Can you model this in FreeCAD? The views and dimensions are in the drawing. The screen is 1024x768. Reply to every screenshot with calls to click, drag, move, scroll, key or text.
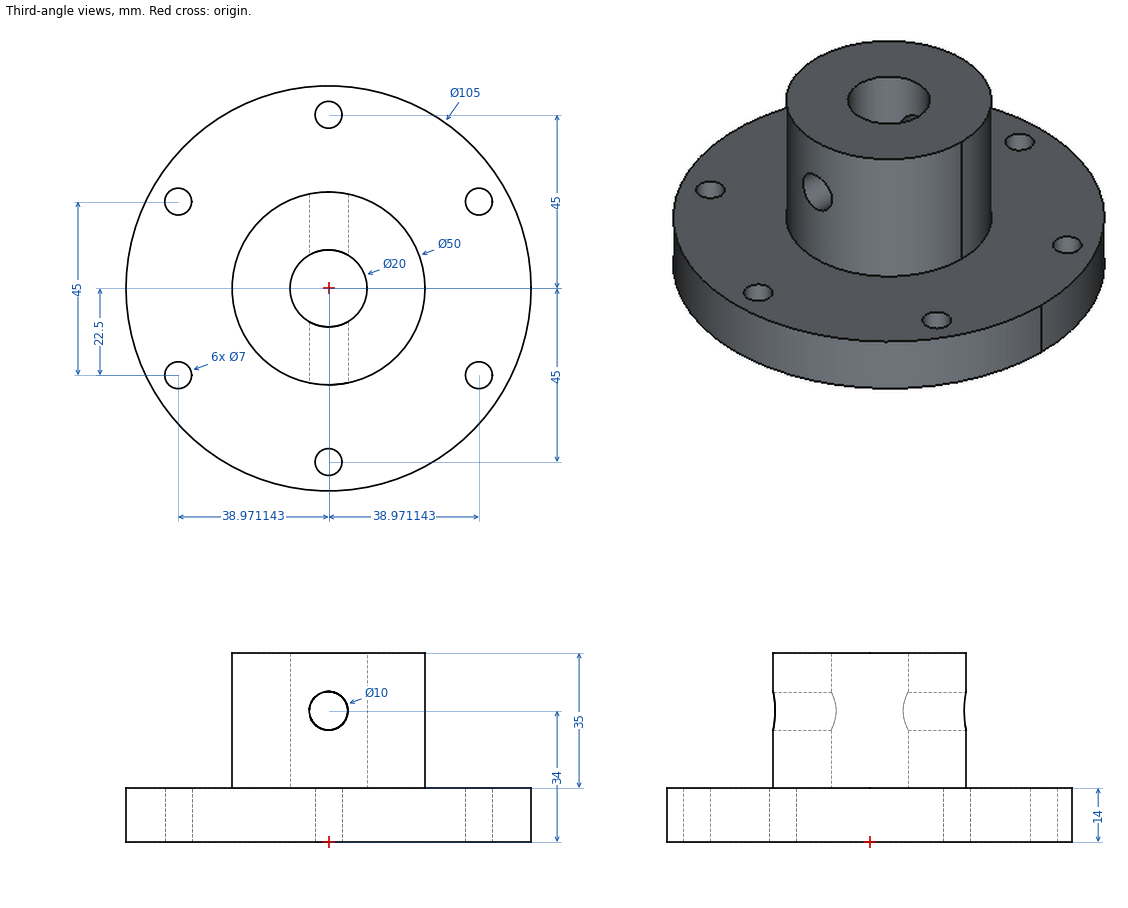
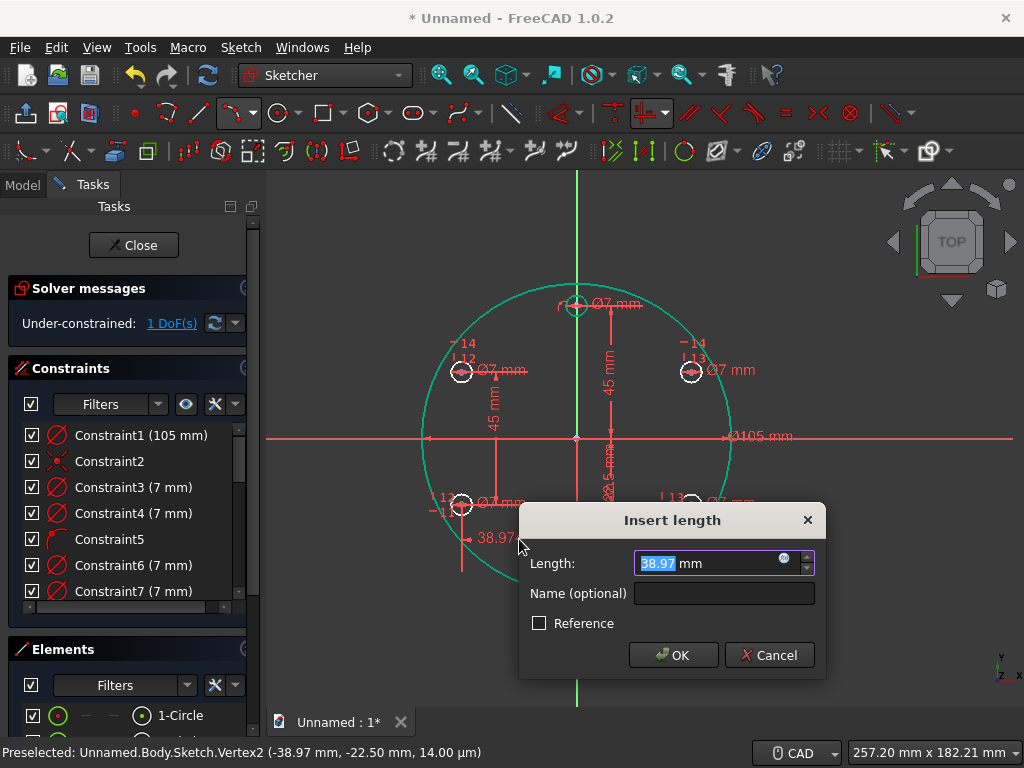
text(38.971143)
key(Return)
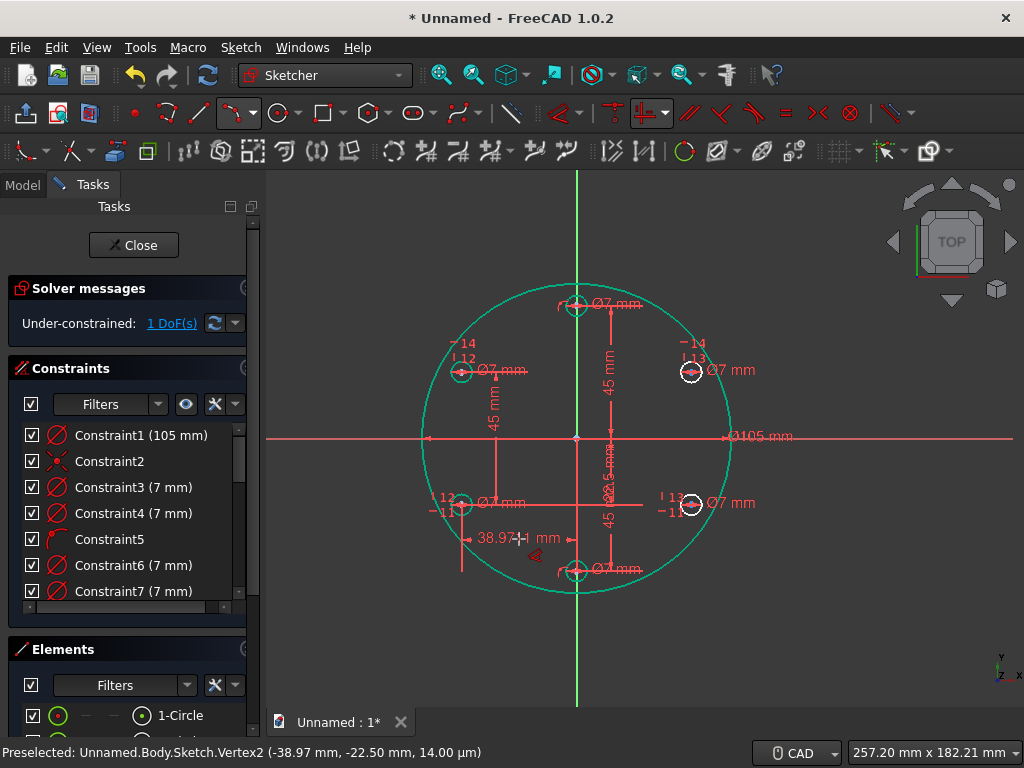
click(691, 505)
click(634, 539)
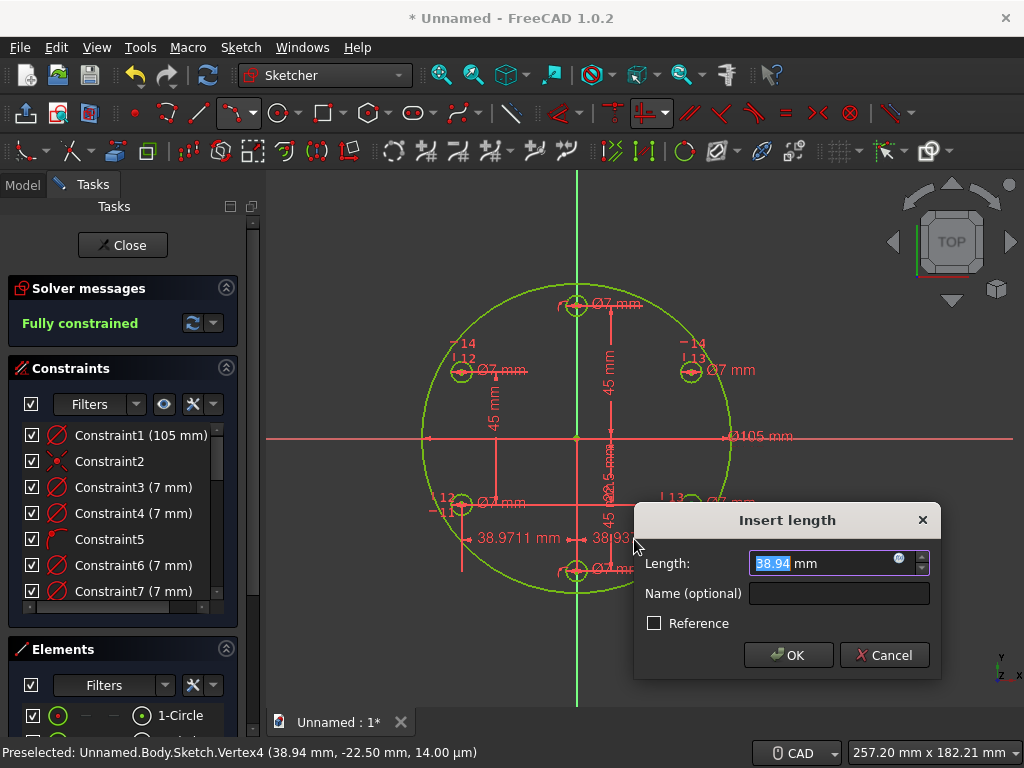
text(38.971143)
key(Return)
key(Escape)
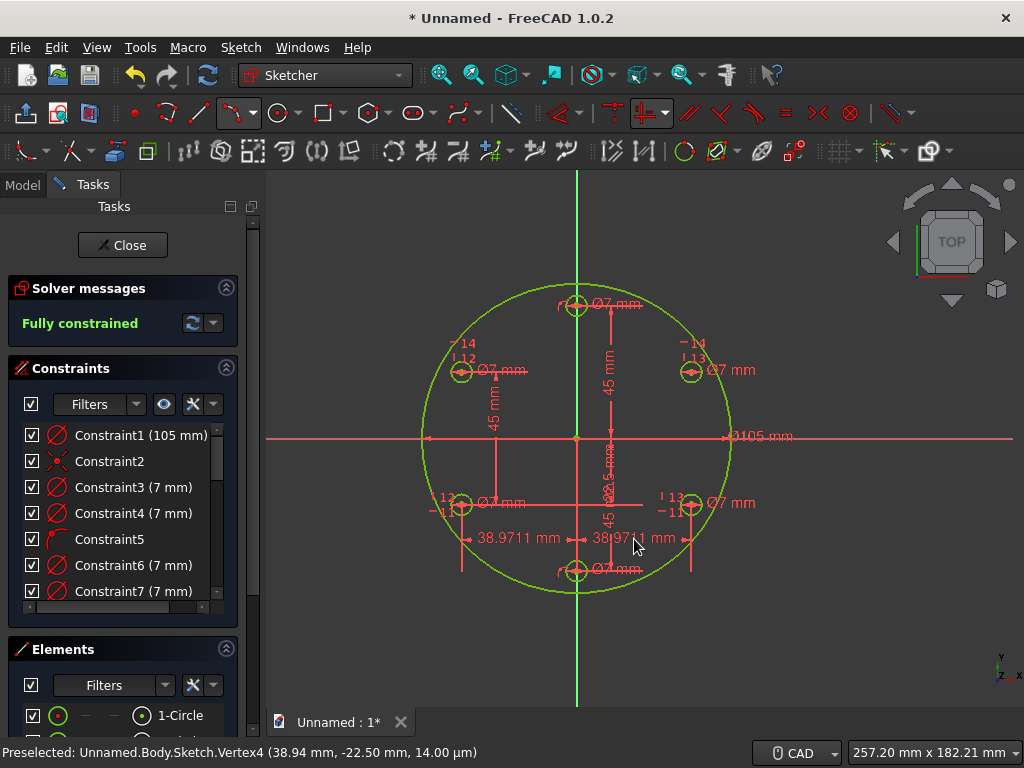
click(123, 245)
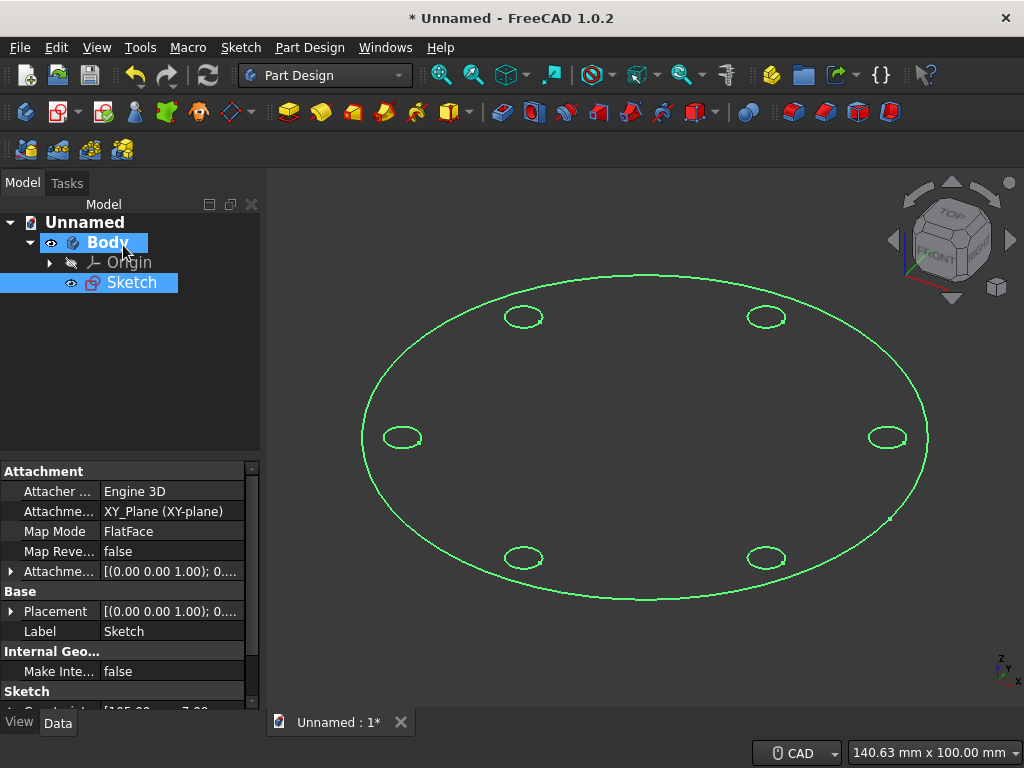
click(290, 112)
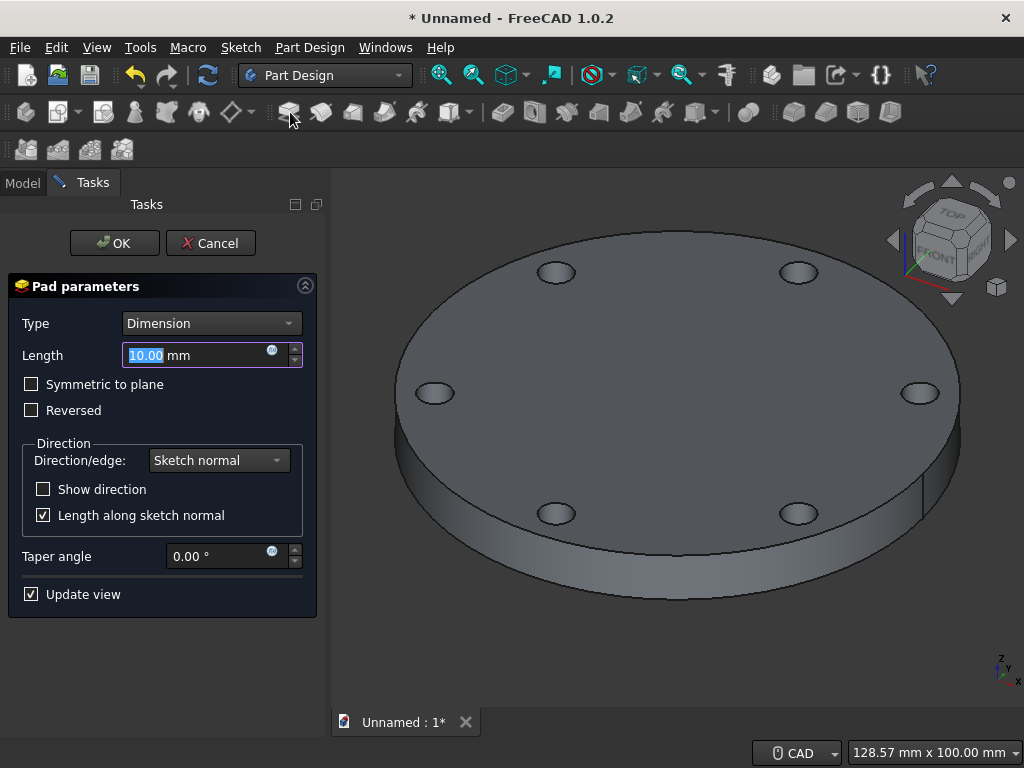
text(14)
key(Tab)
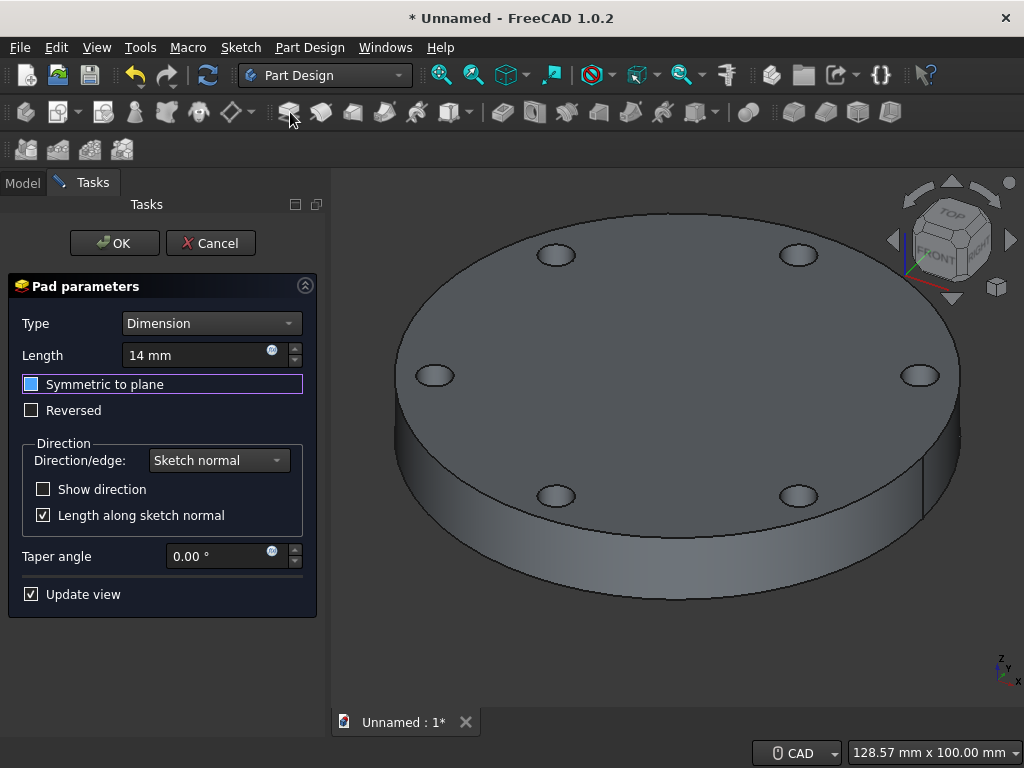
click(115, 243)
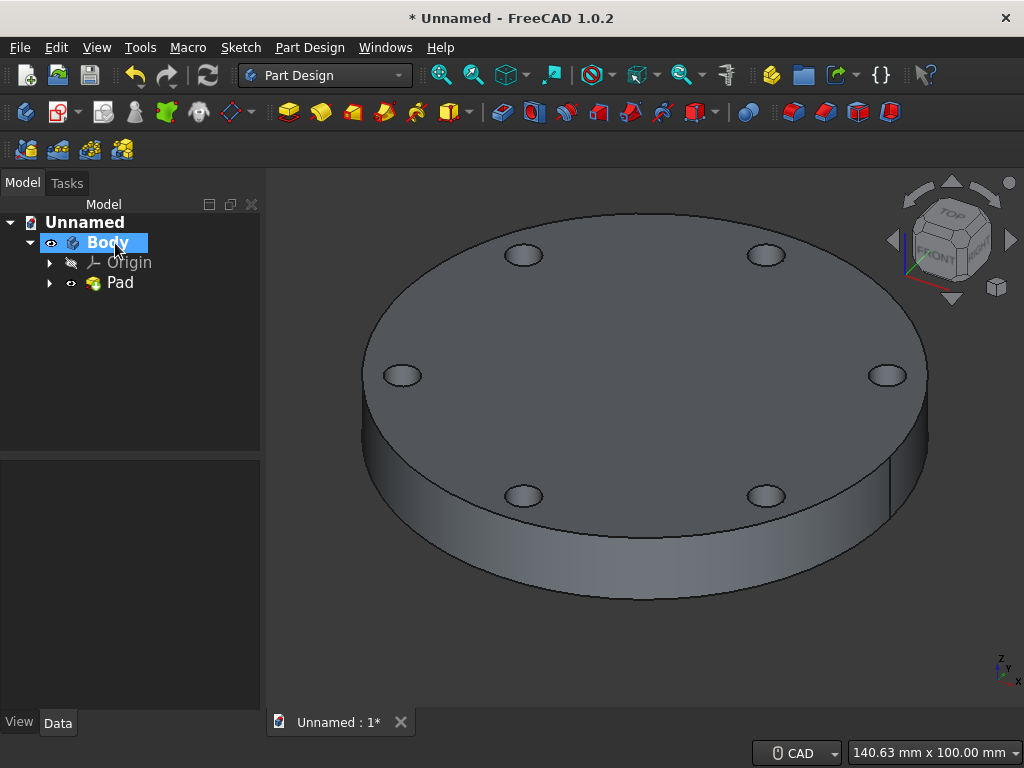
key(v)
key(f)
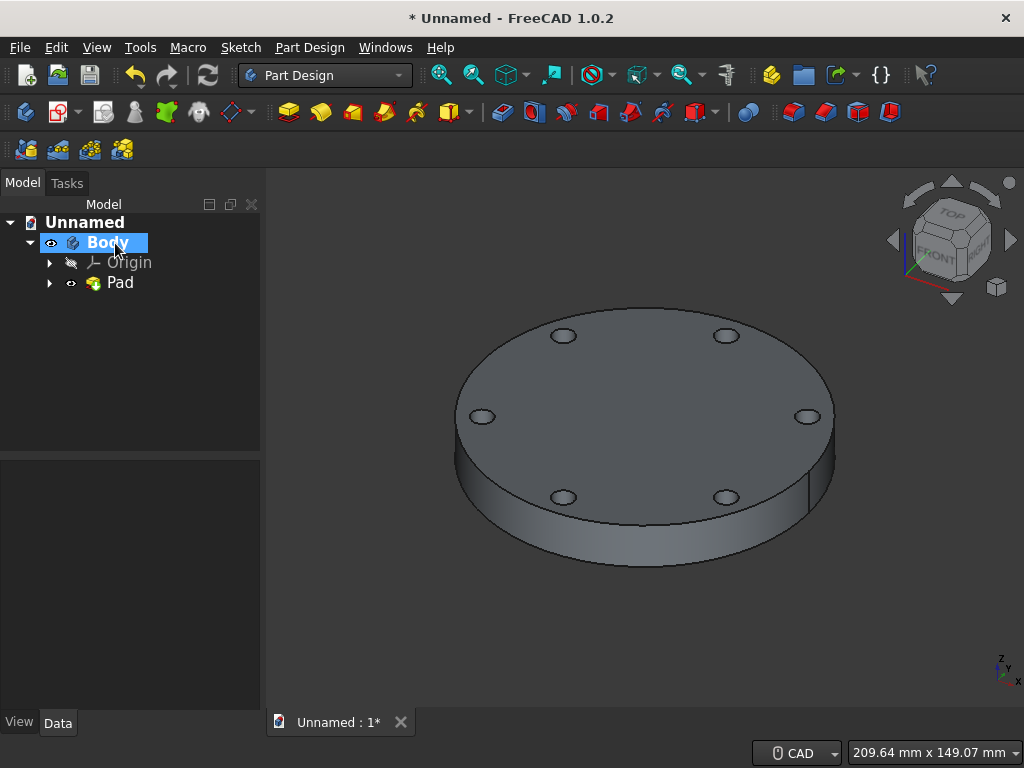
click(645, 416)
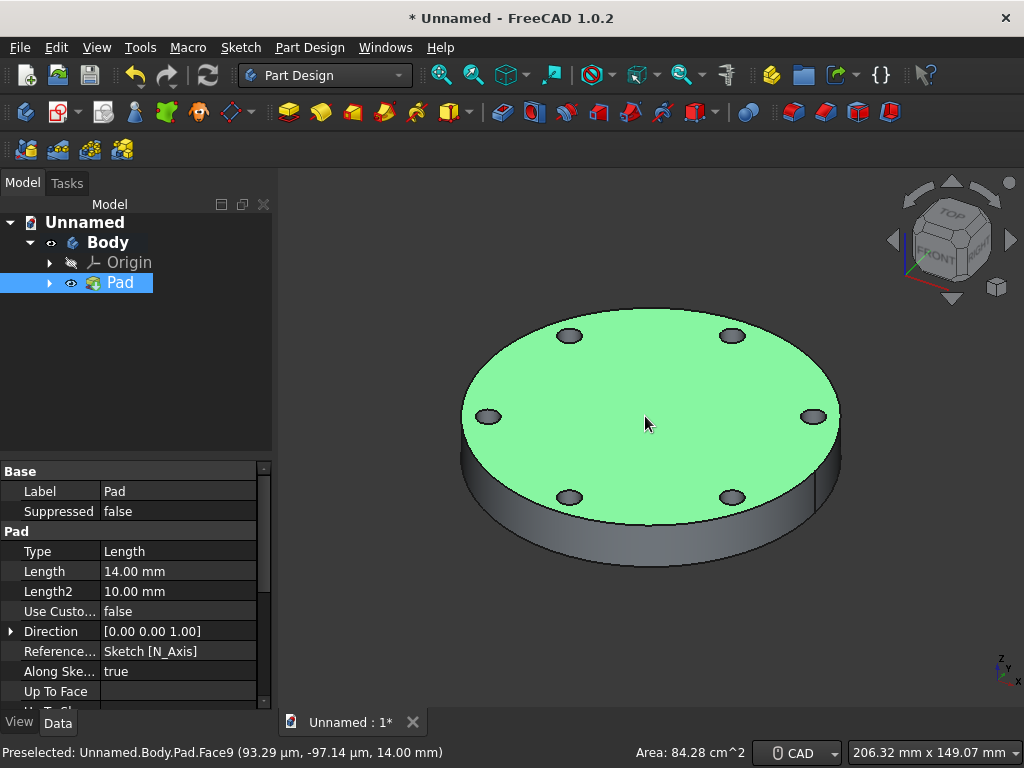
click(58, 112)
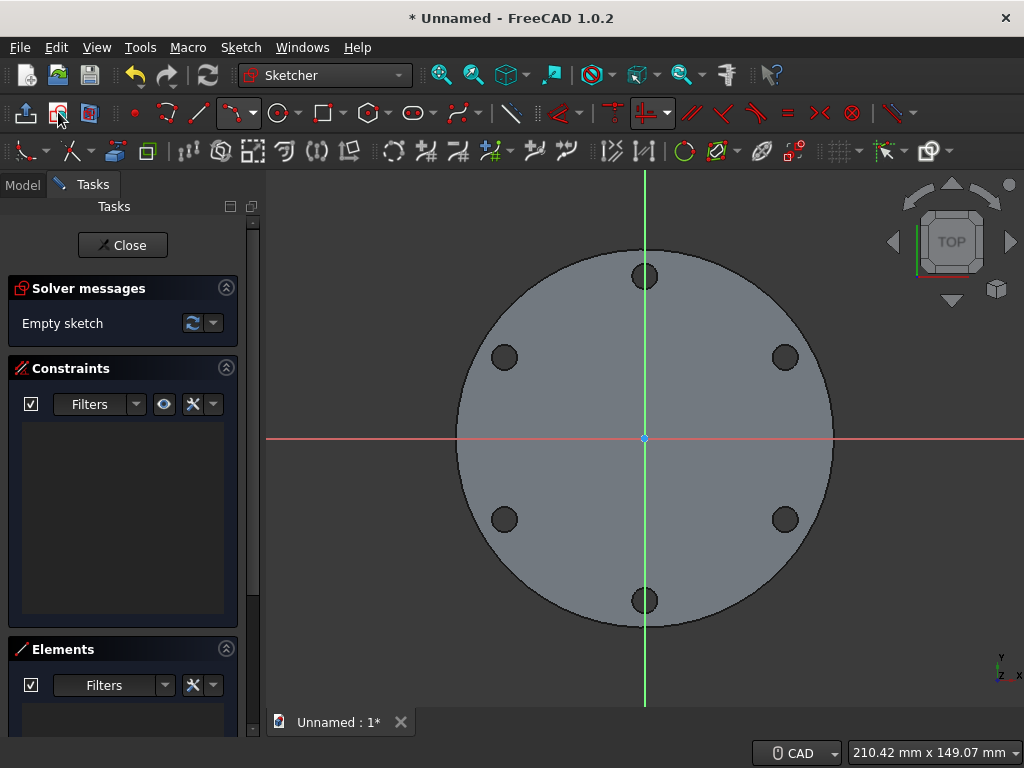
scroll(728, 438, up, 3)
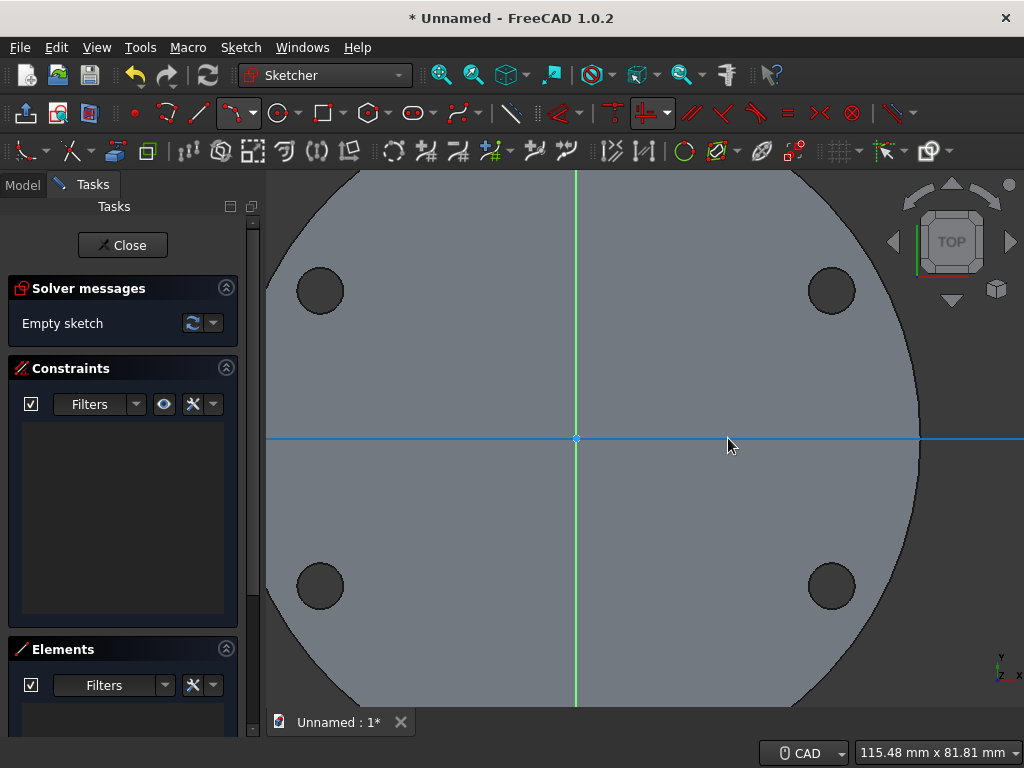
key(g)
key(c)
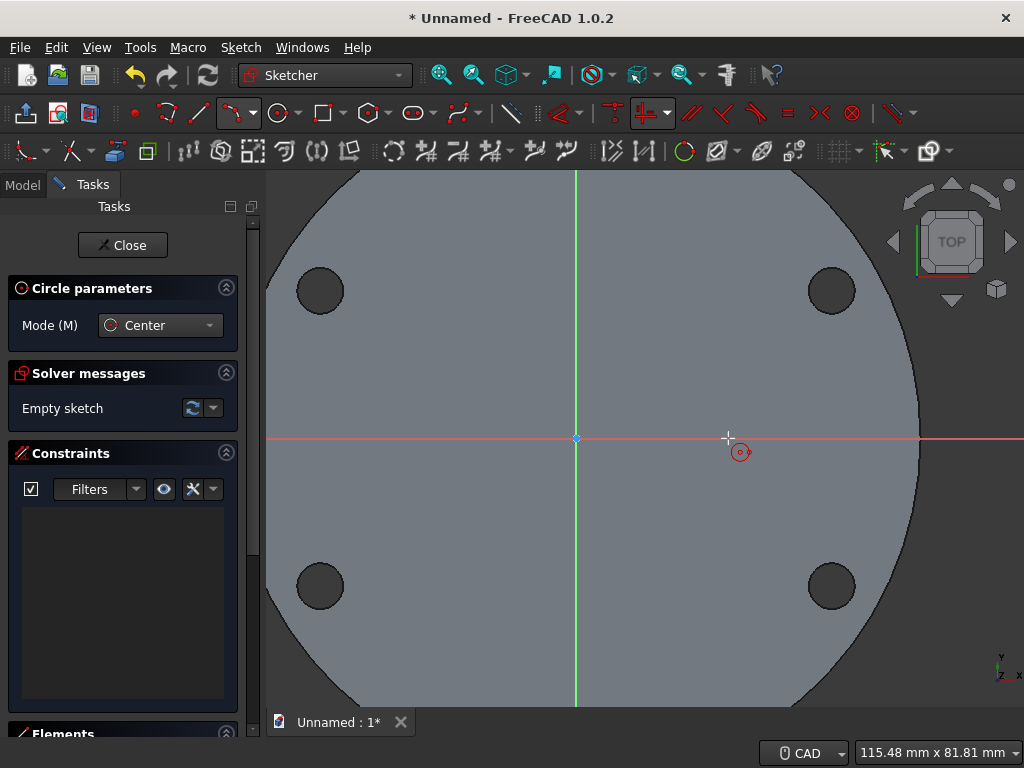
click(576, 438)
move(692, 322)